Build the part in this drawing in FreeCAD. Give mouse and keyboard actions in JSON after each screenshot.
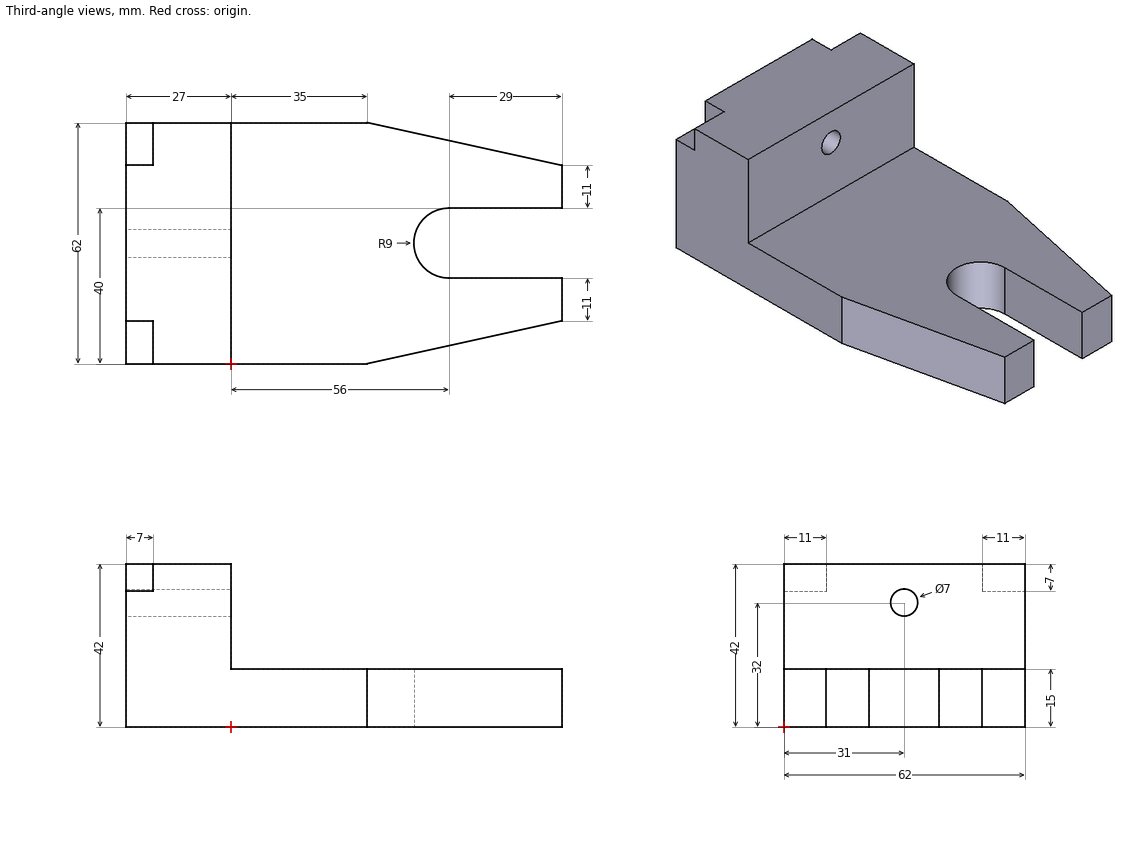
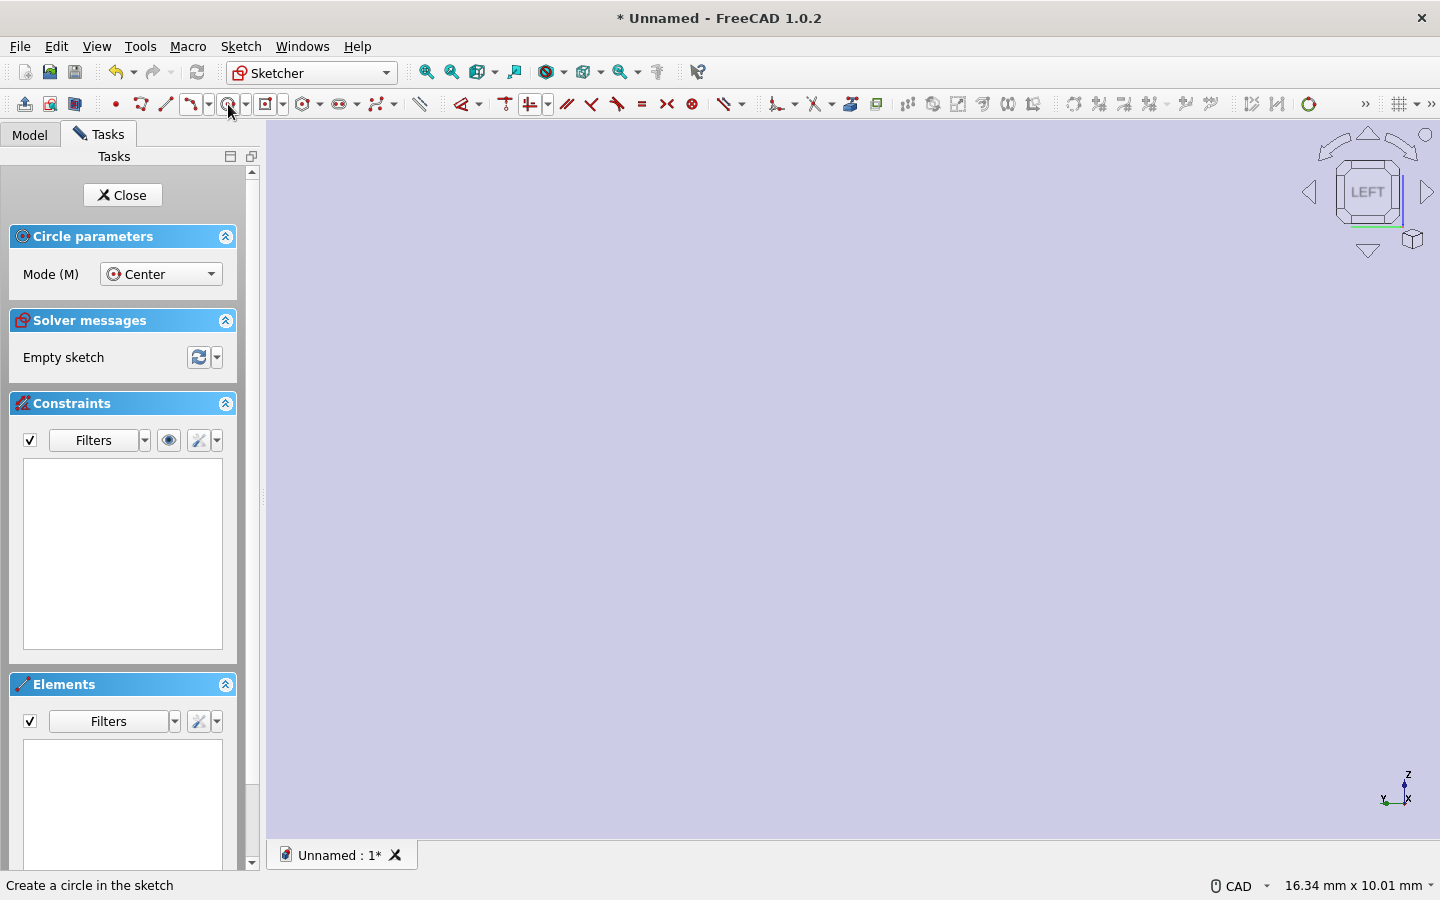
{"action": "left_click", "coordinate": [784, 475]}
{"action": "left_click", "coordinate": [962, 298]}
{"action": "key", "text": "Escape"}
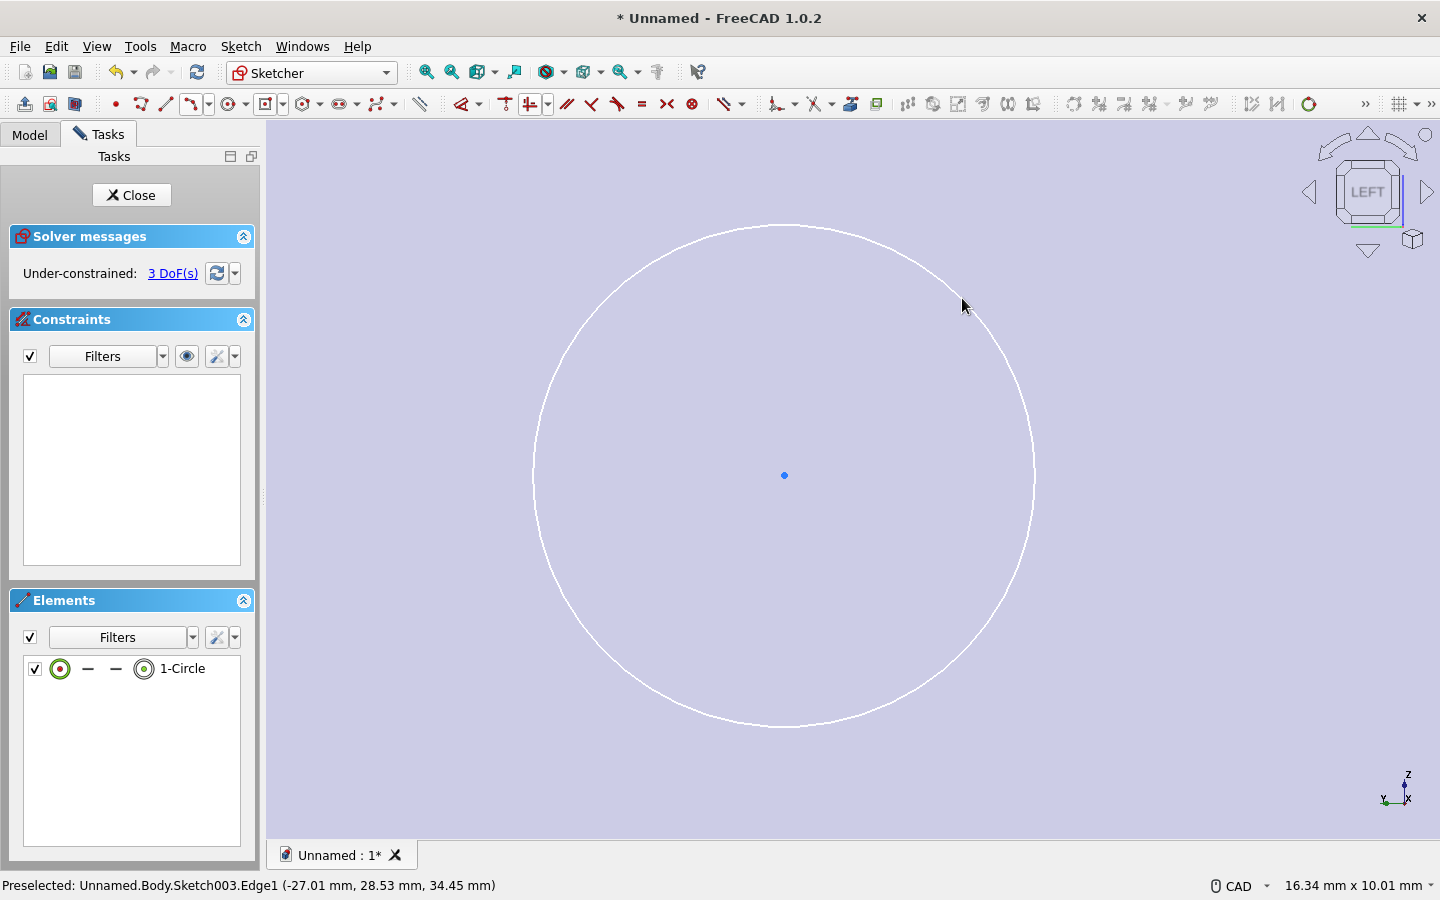
{"action": "left_click", "coordinate": [460, 104]}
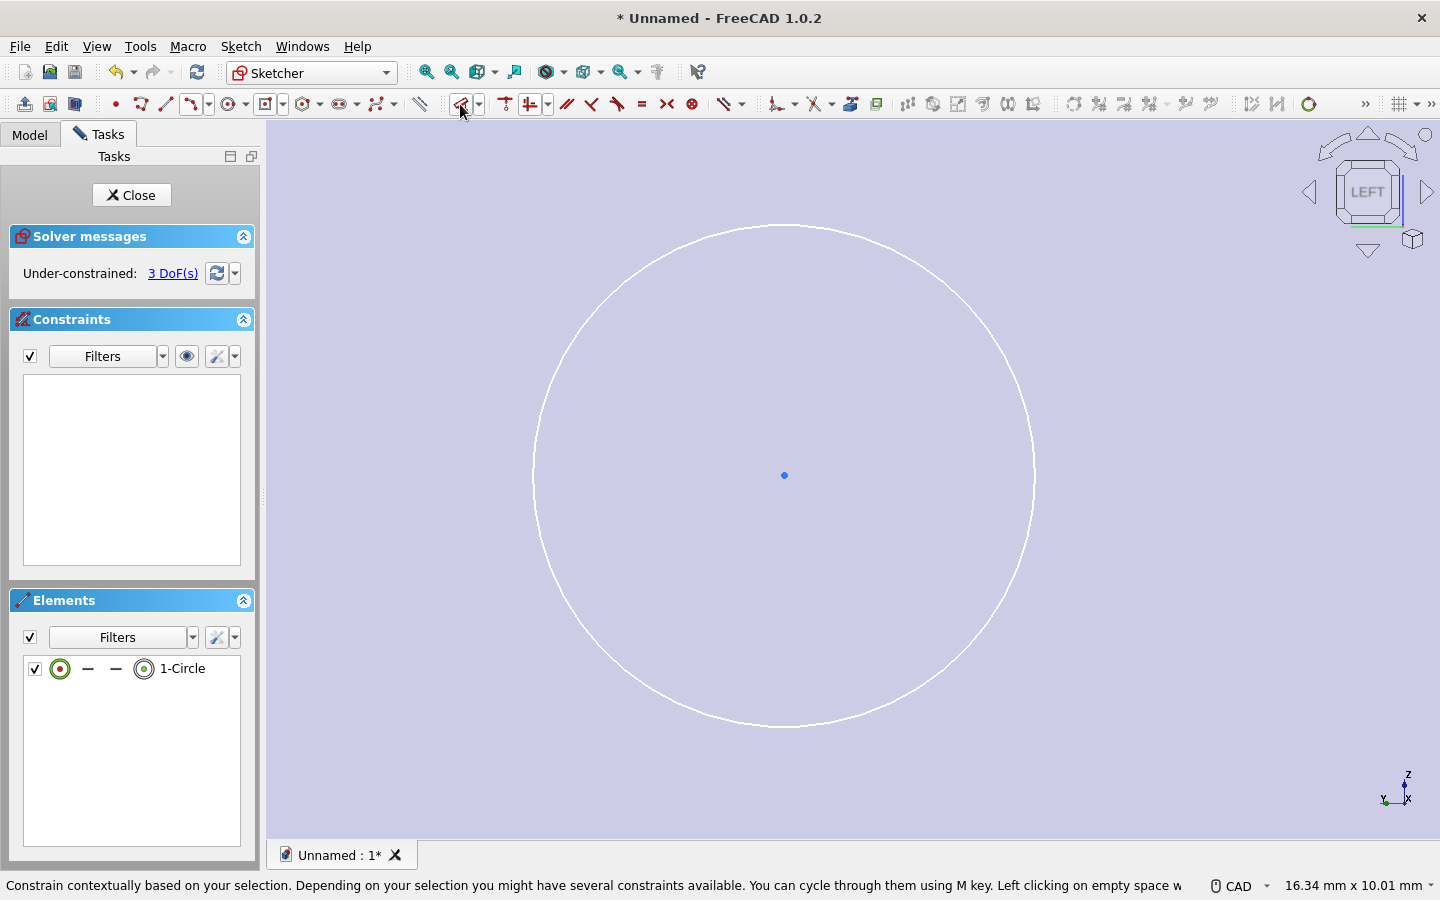
{"action": "left_click", "coordinate": [961, 298]}
{"action": "left_click", "coordinate": [984, 275]}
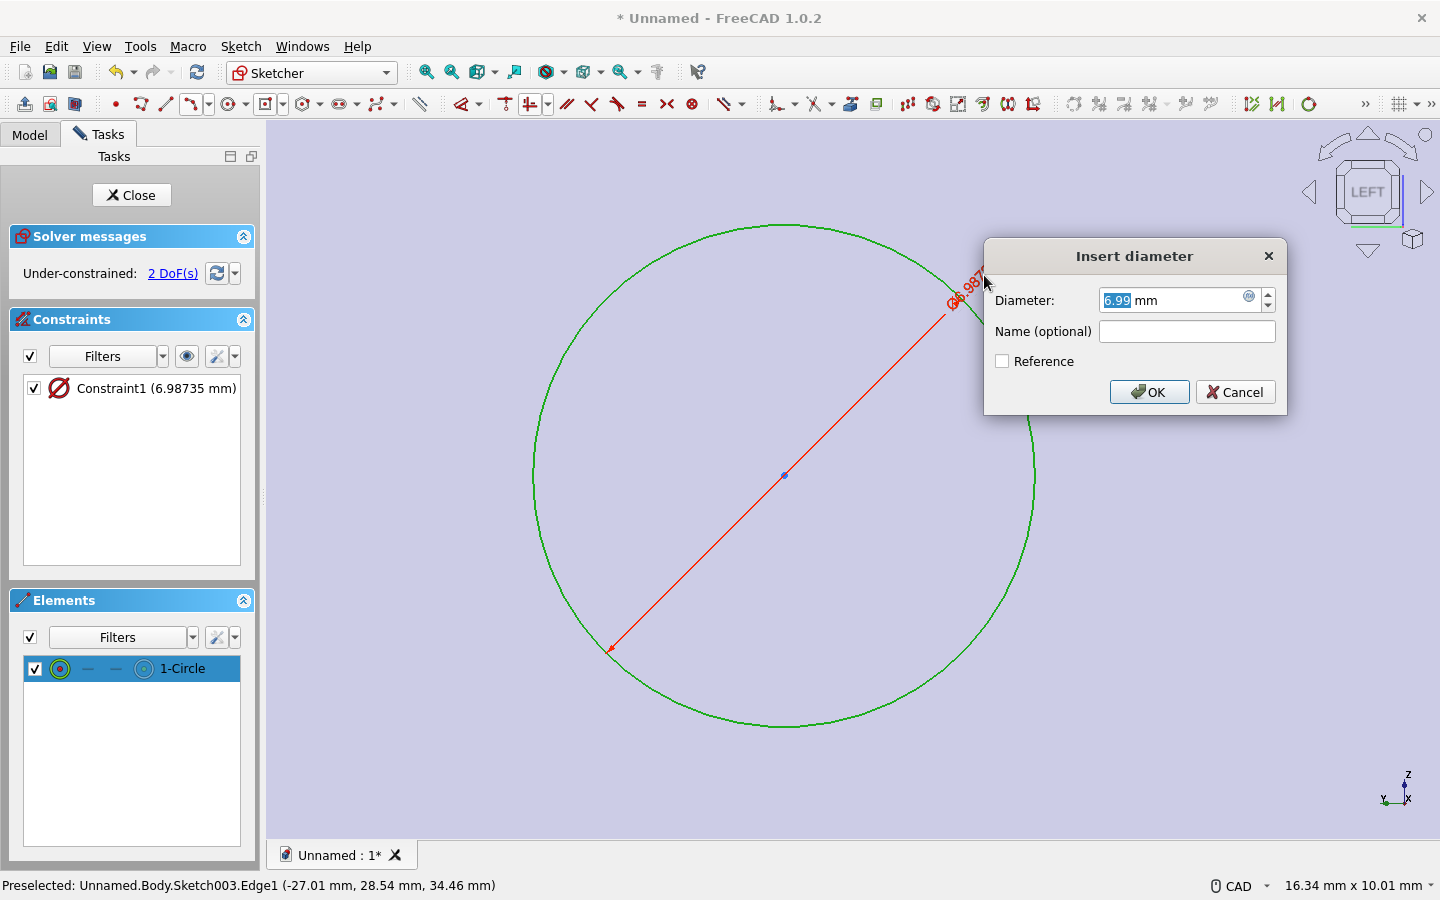
{"action": "type", "text": "7"}
{"action": "key", "text": "Return"}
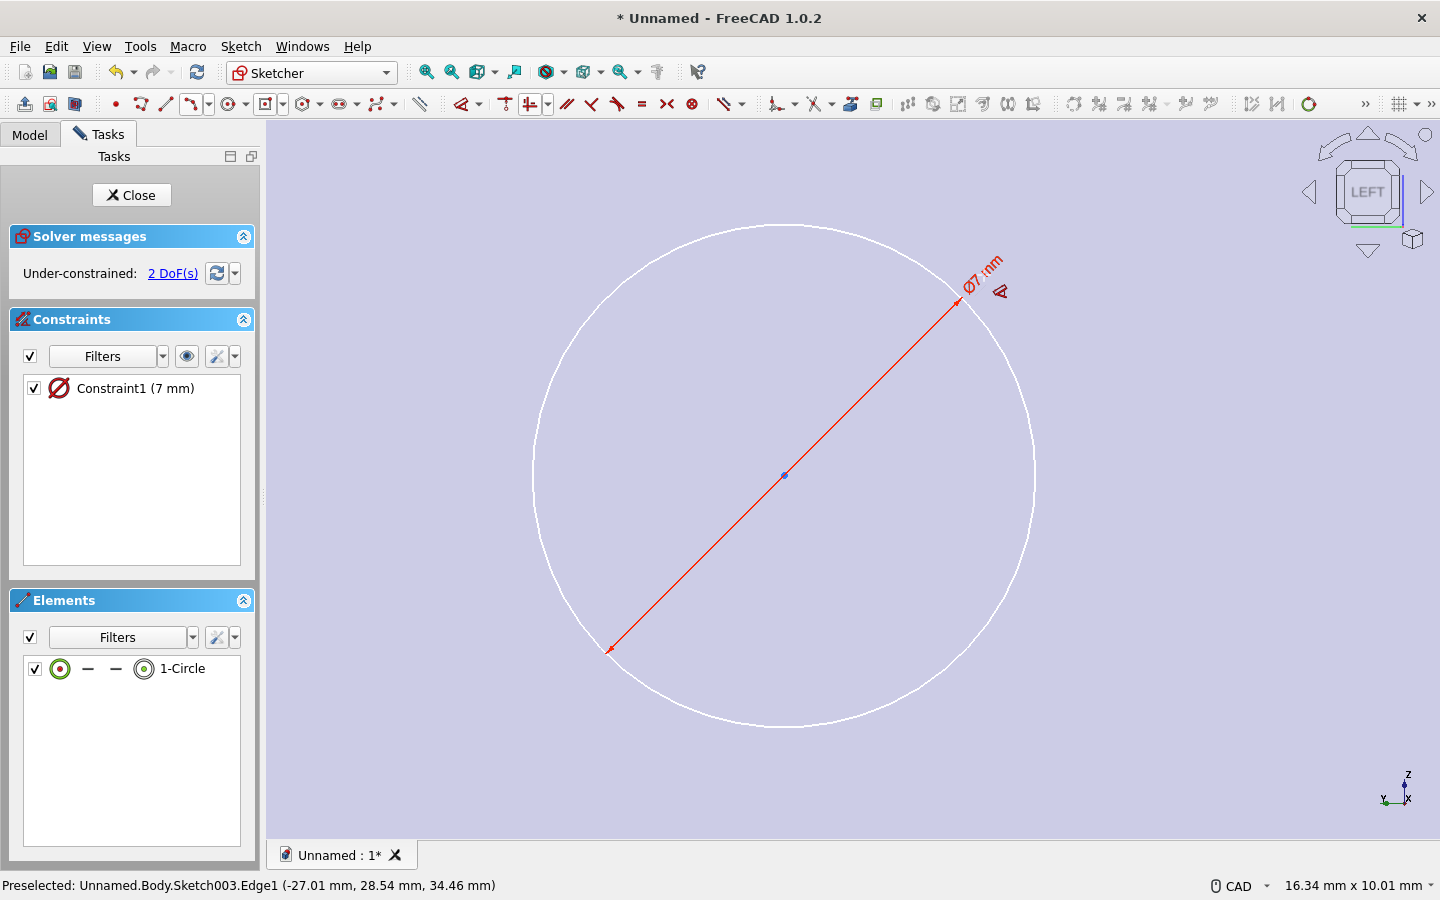
{"action": "left_click", "coordinate": [784, 476]}
{"action": "left_click", "coordinate": [917, 442]}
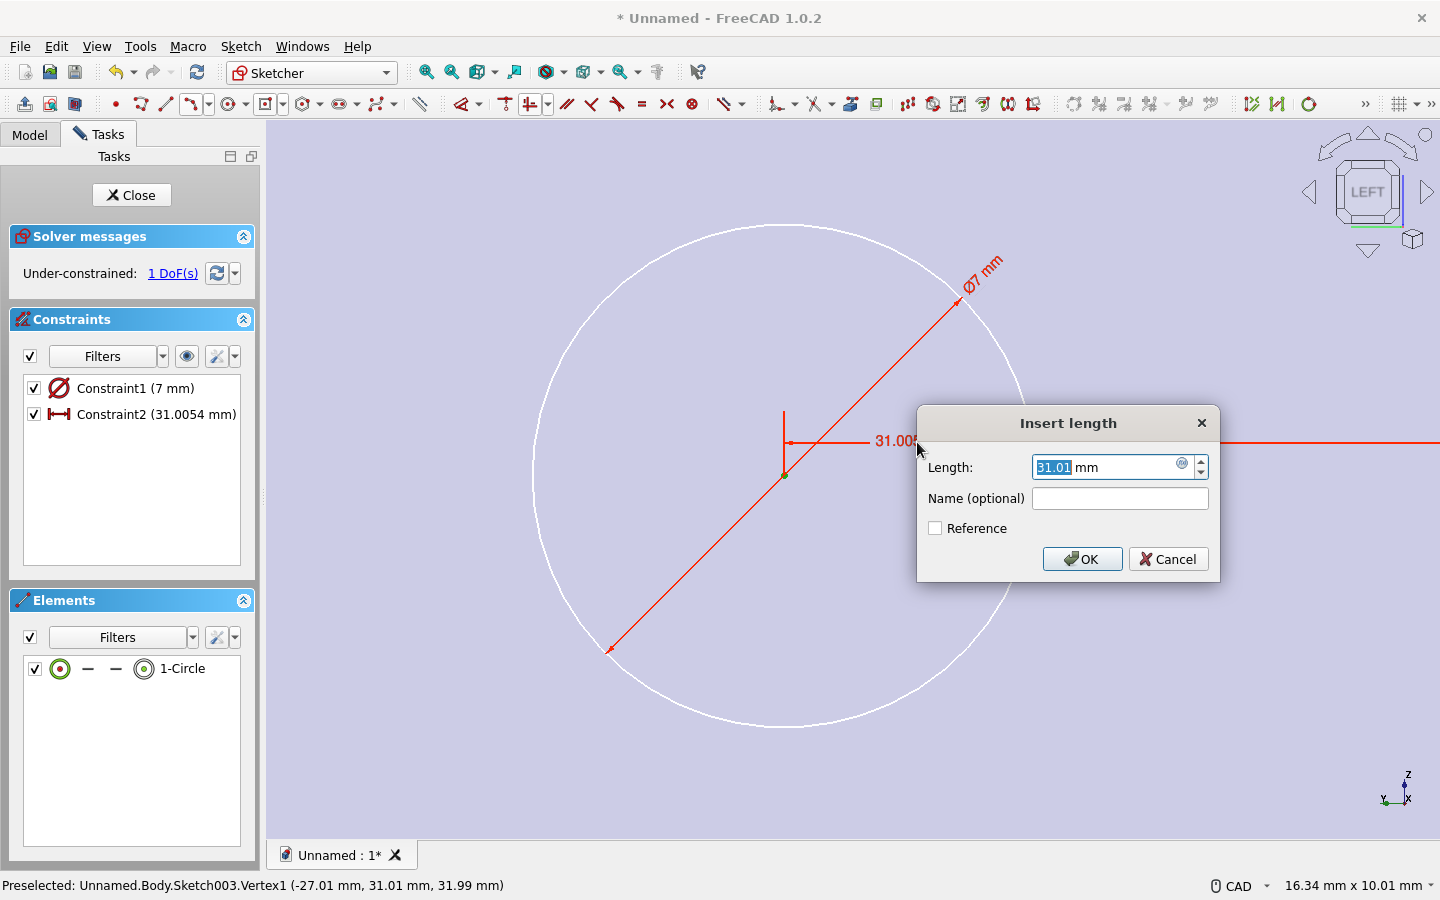
{"action": "type", "text": "31"}
{"action": "key", "text": "Return"}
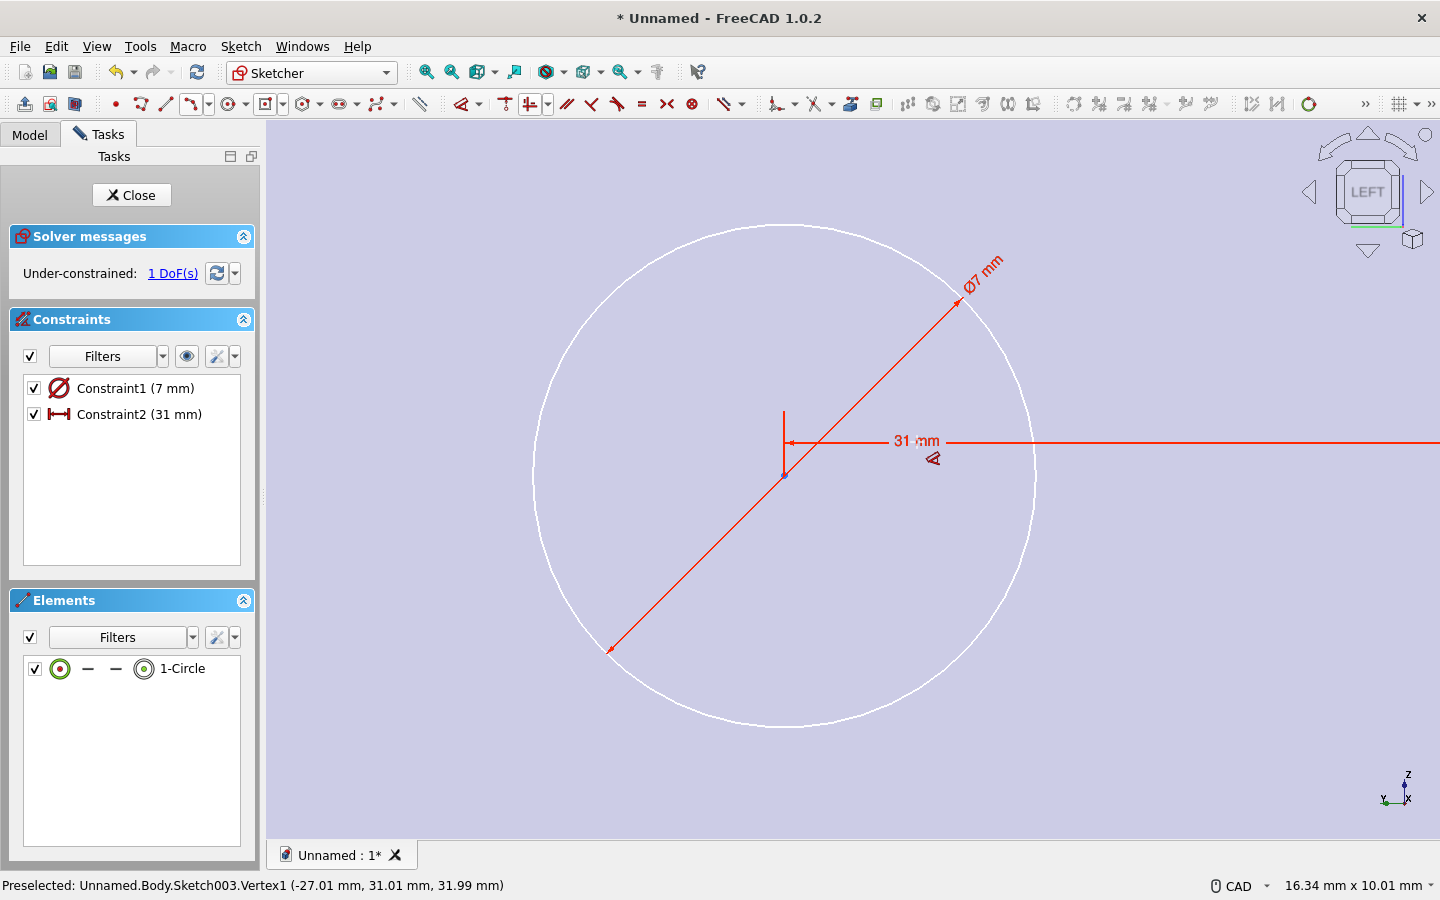
{"action": "left_click", "coordinate": [784, 476]}
{"action": "left_click", "coordinate": [750, 644]}